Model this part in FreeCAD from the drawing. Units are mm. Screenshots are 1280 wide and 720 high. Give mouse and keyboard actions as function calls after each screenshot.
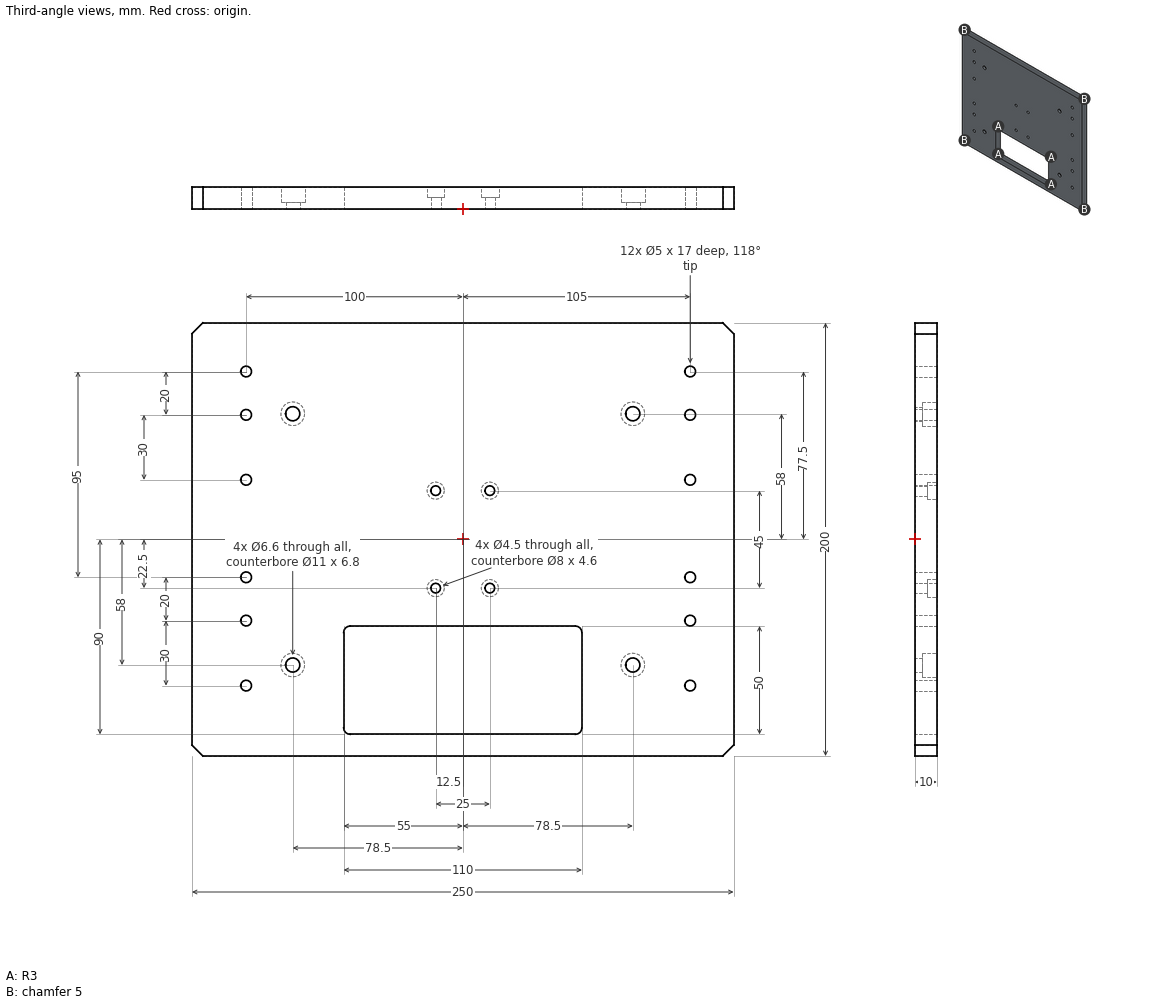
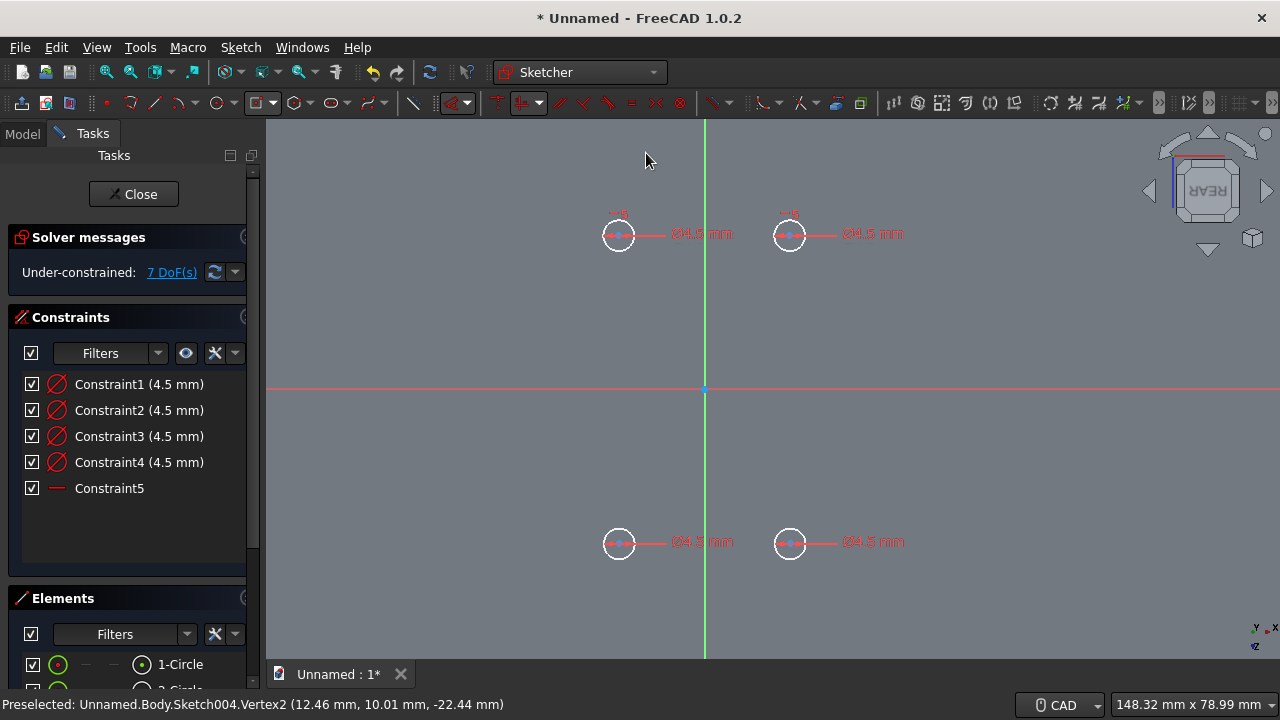
click(790, 236)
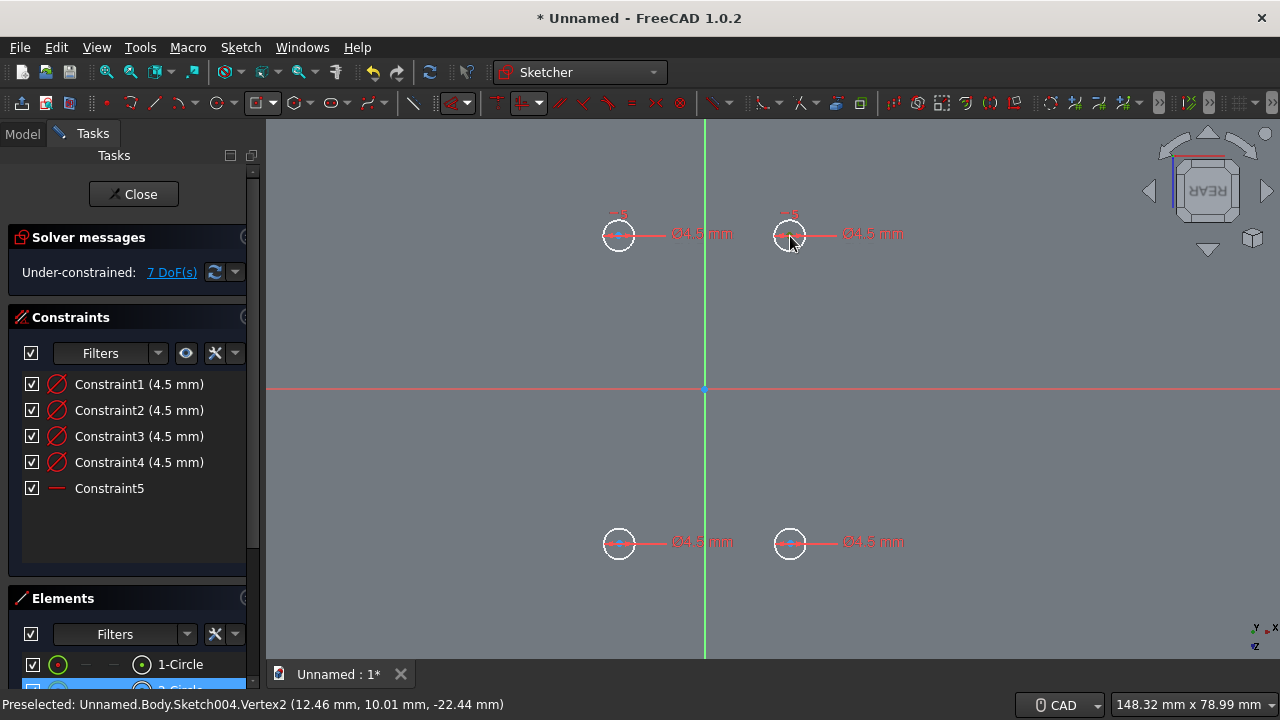
click(790, 544)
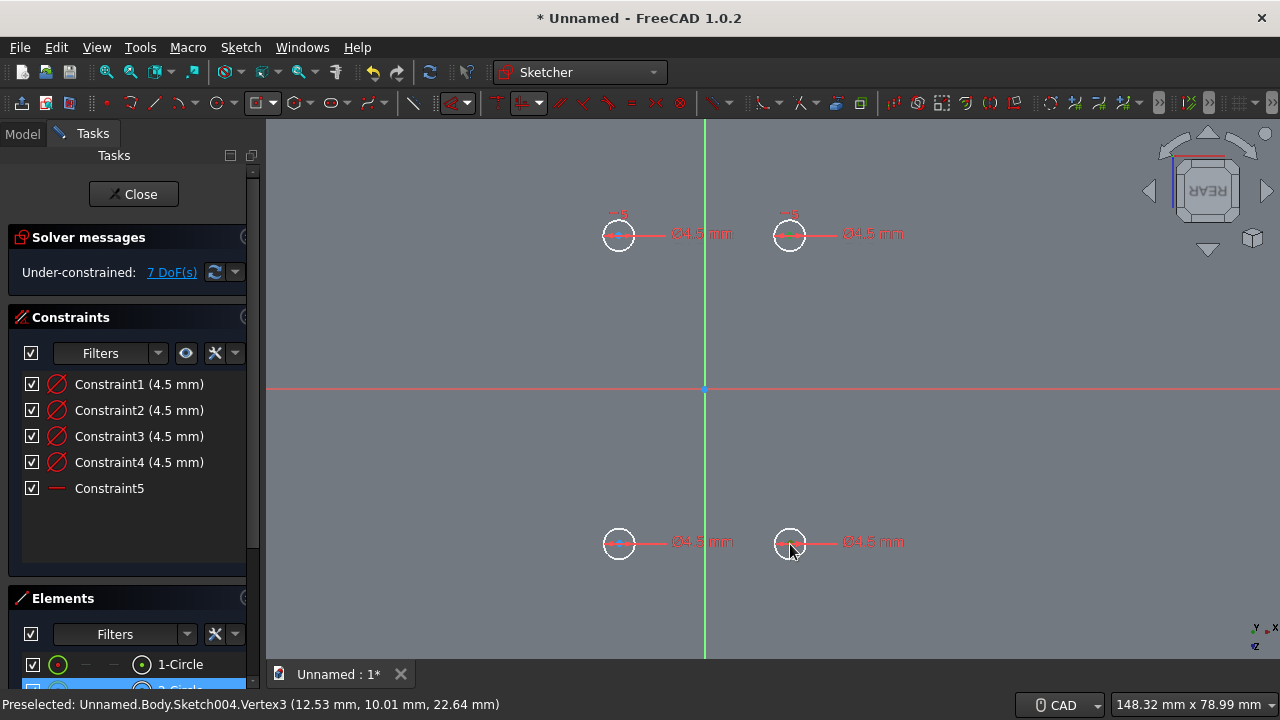
click(542, 104)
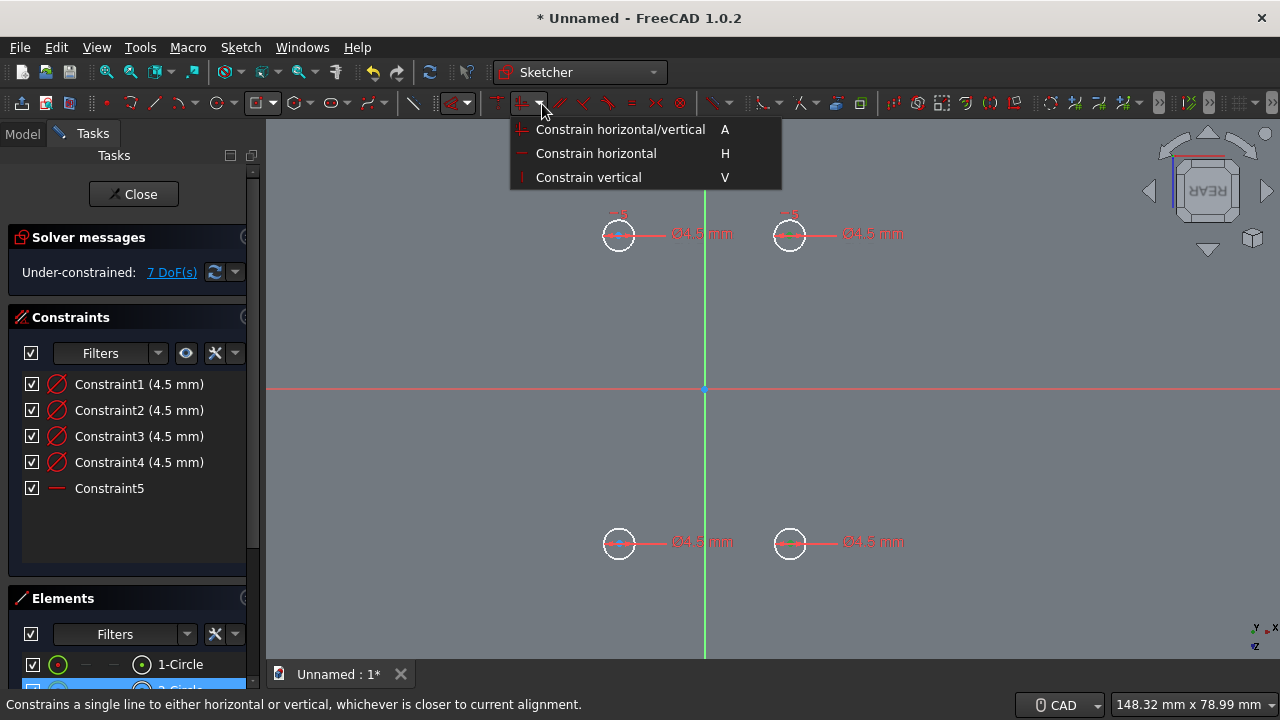
click(646, 177)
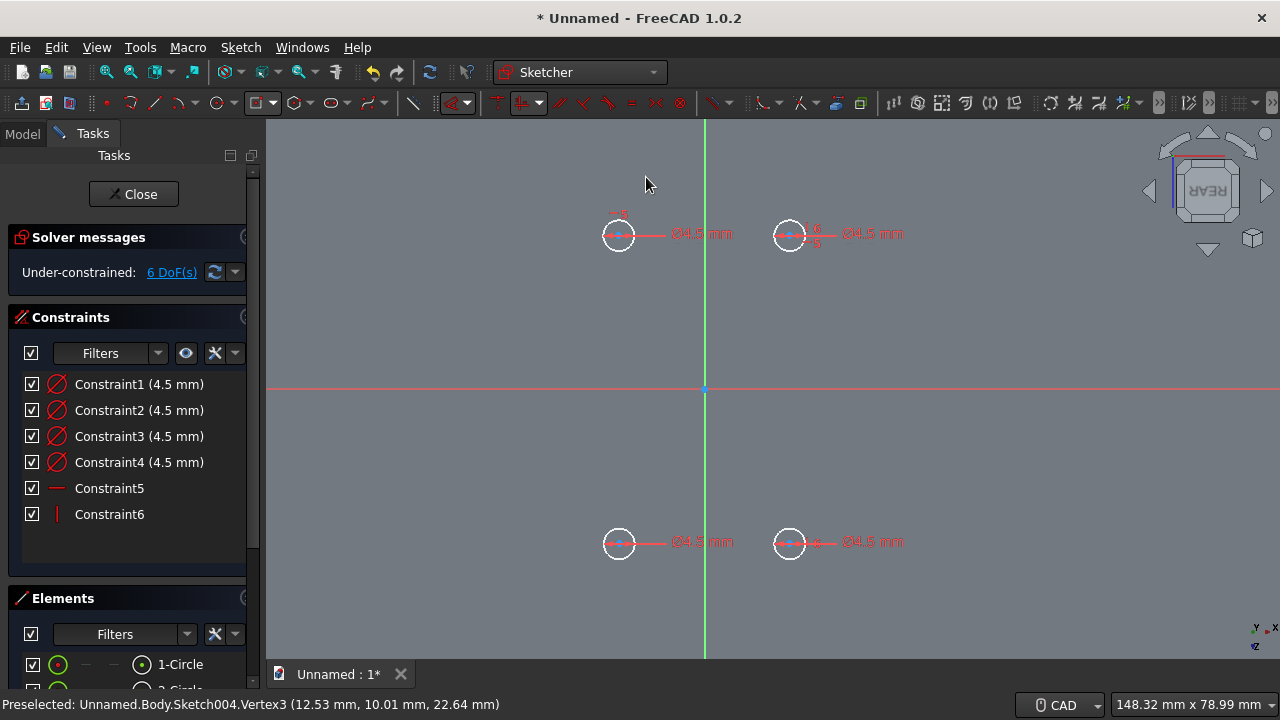
click(619, 236)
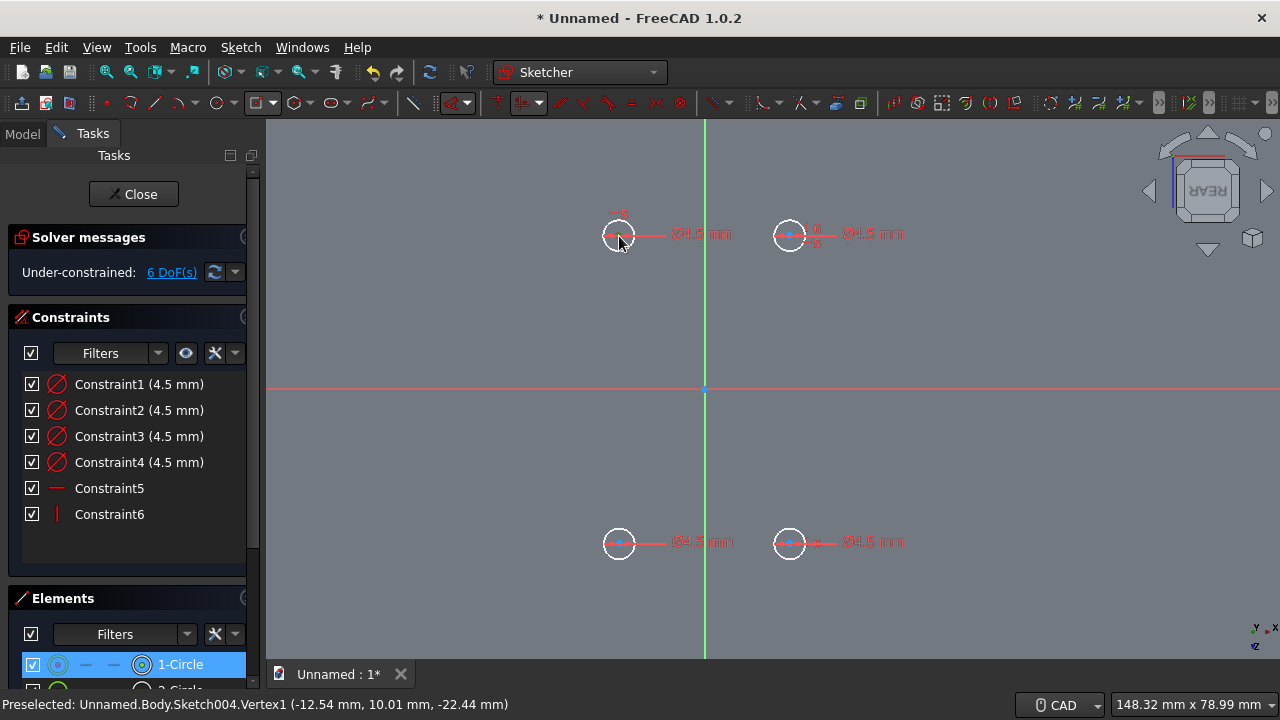
click(619, 544)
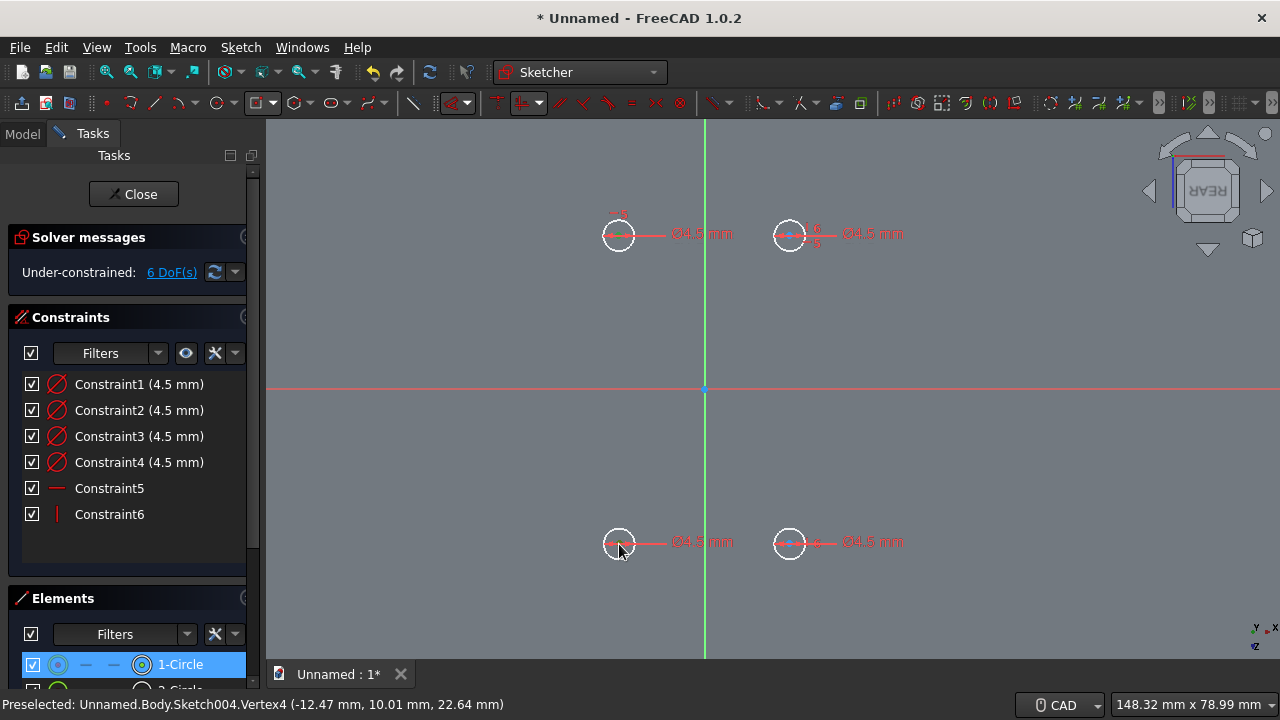
click(542, 104)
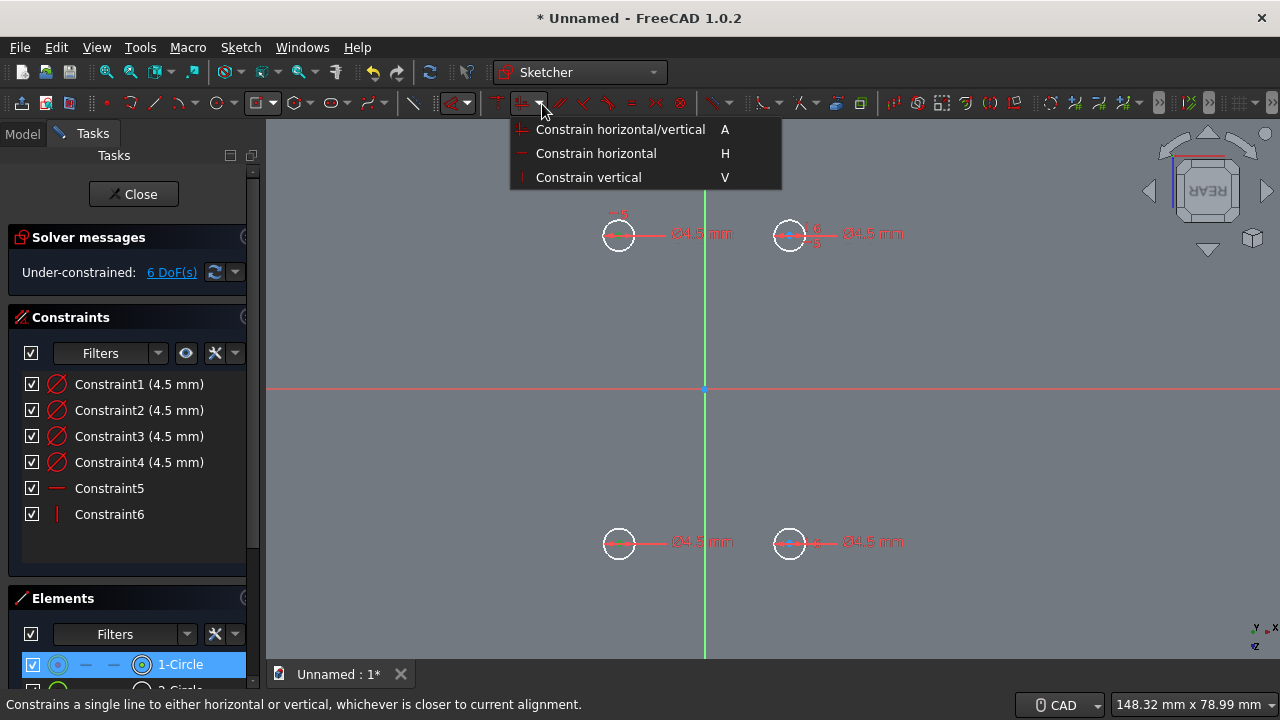
click(646, 177)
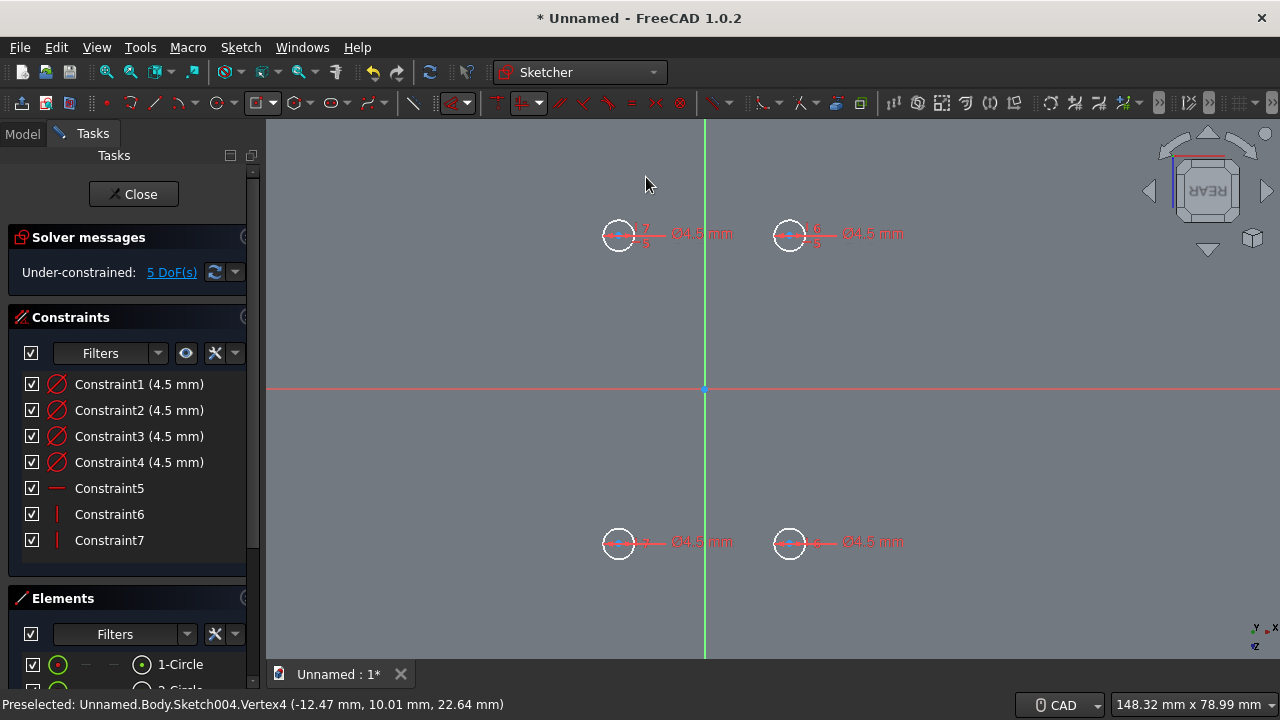
click(790, 544)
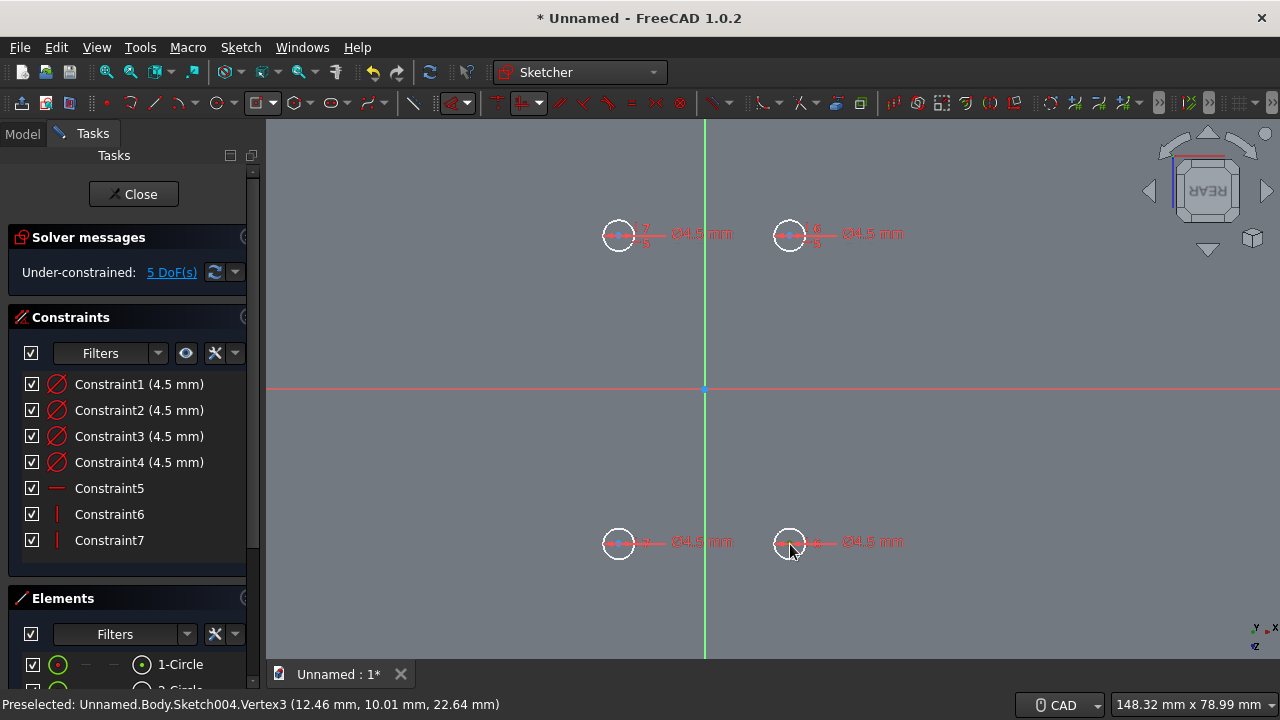
click(619, 544)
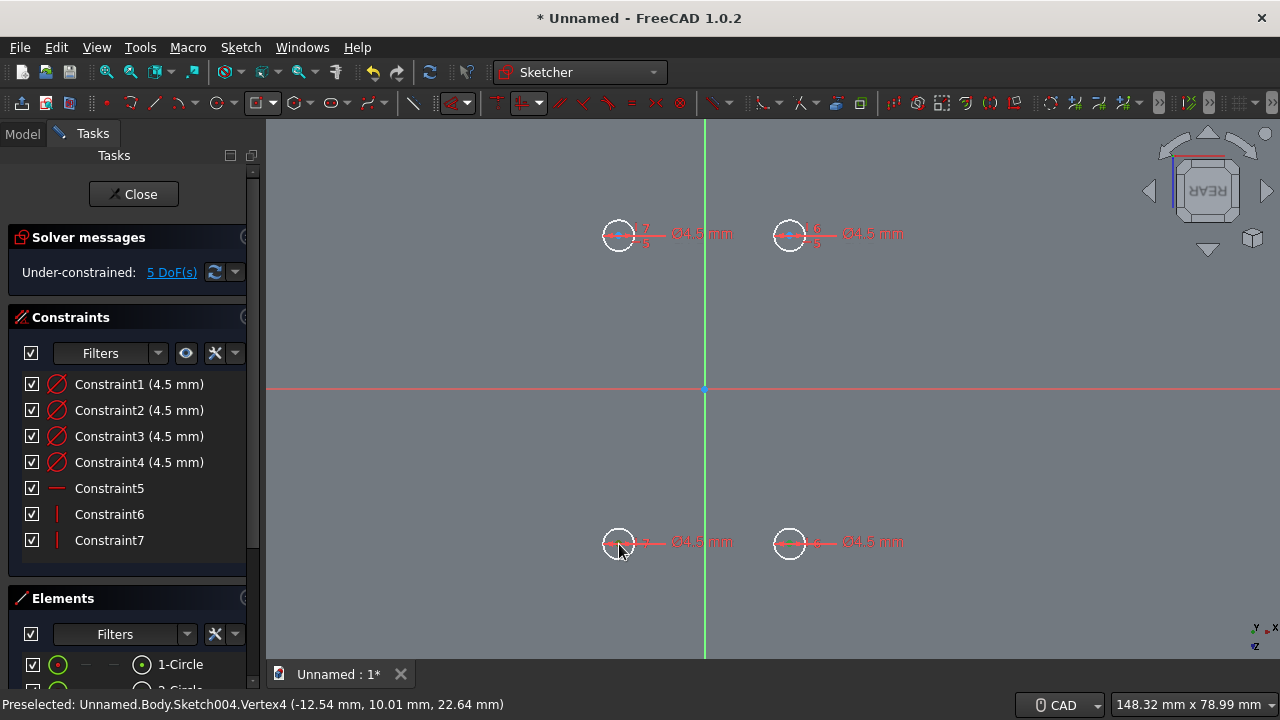
click(542, 104)